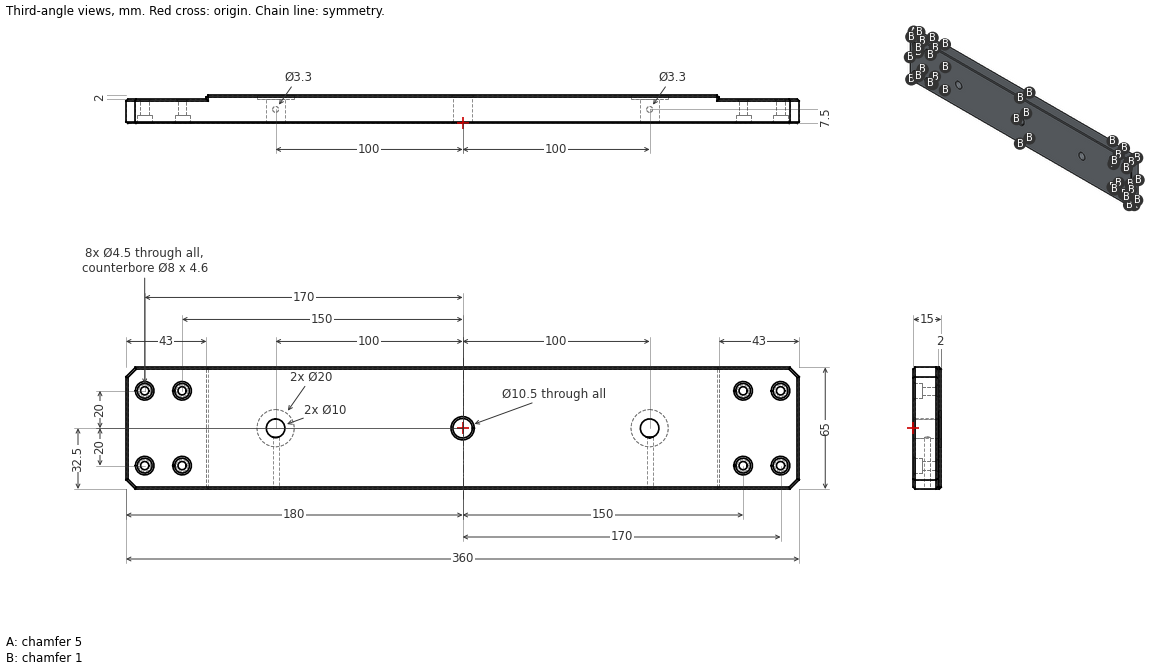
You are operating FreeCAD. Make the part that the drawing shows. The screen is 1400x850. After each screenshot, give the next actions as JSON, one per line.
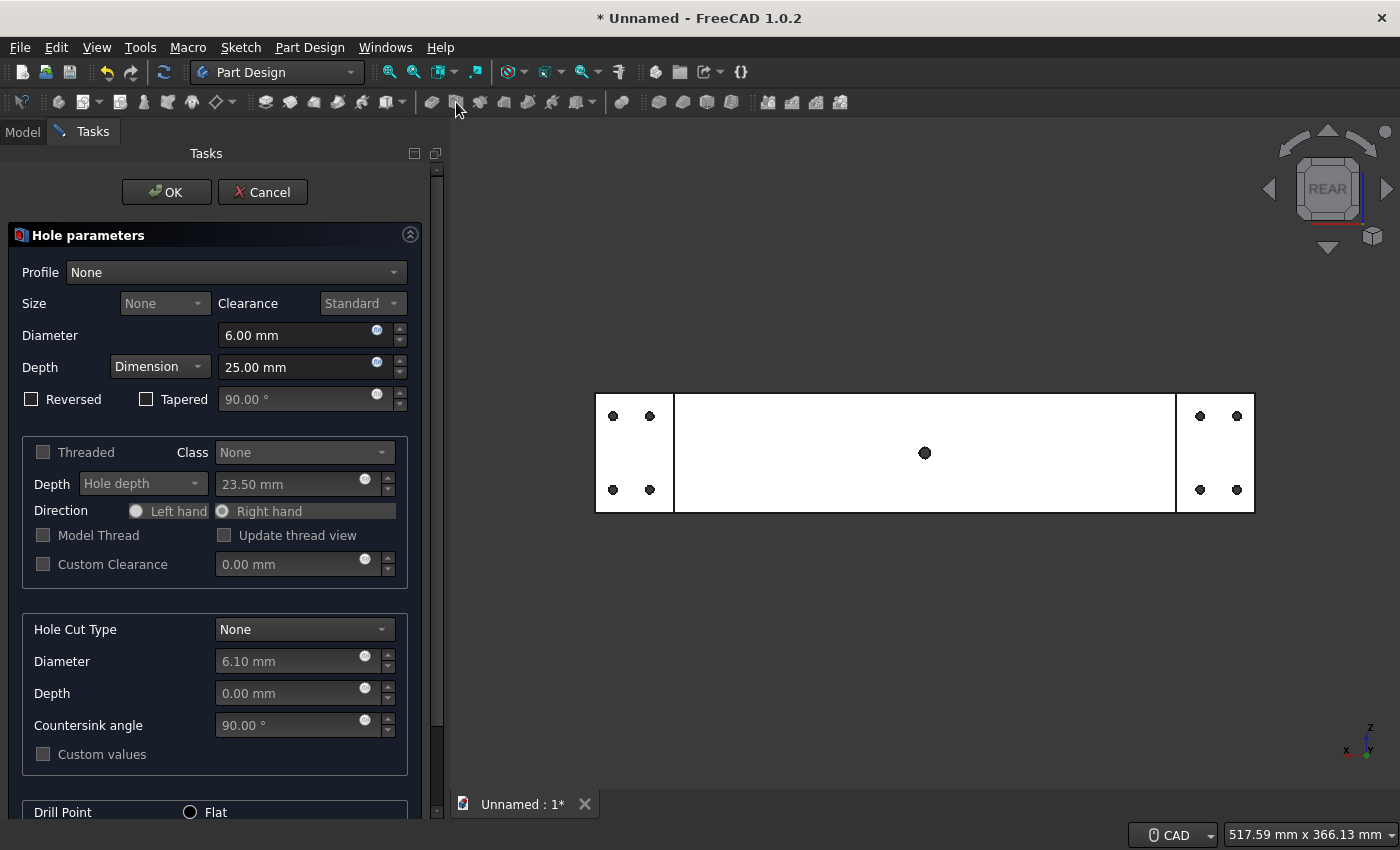
{"action": "triple_click", "coordinate": [305, 335]}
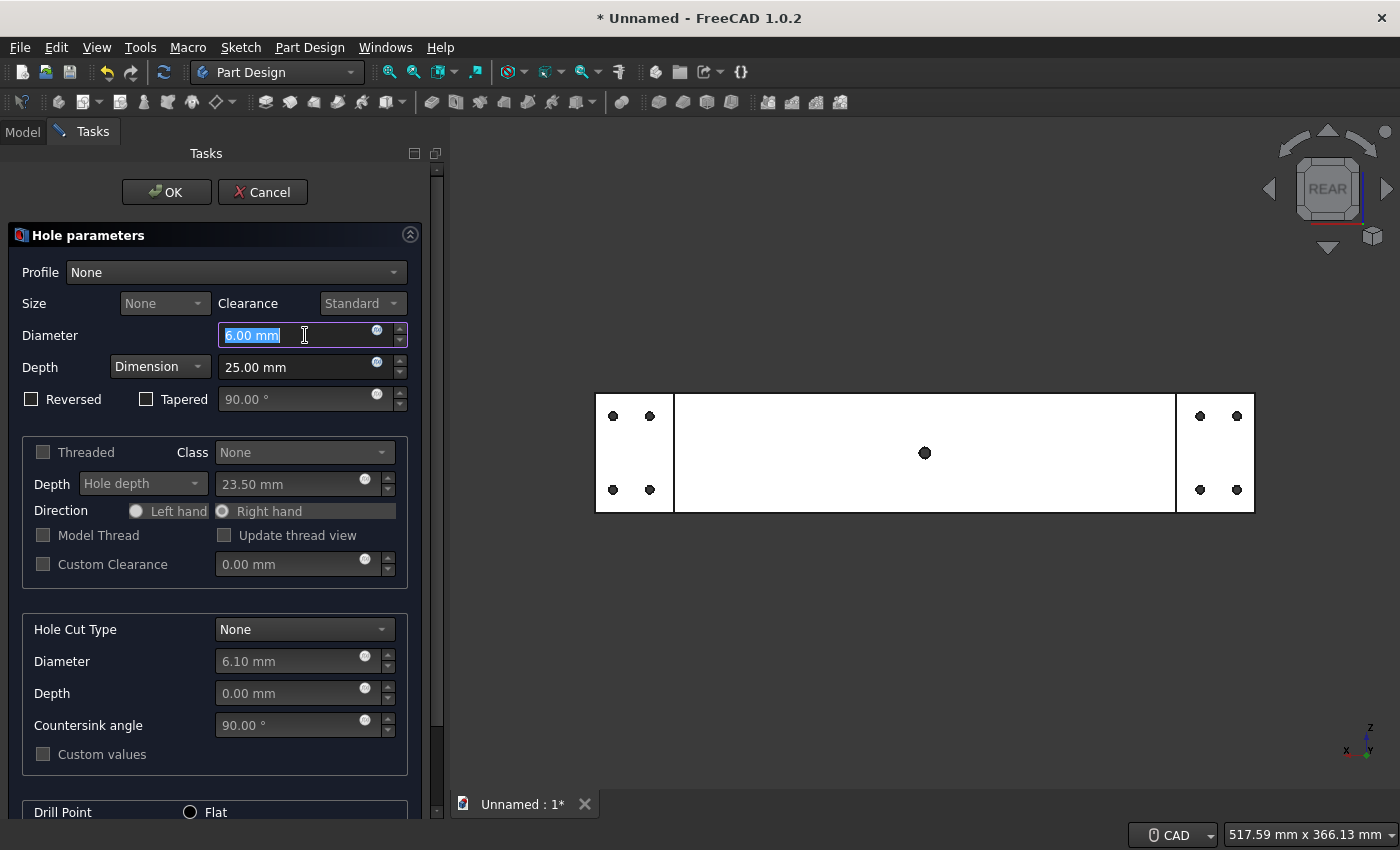
{"action": "type", "text": "10.5"}
{"action": "key", "text": "Tab"}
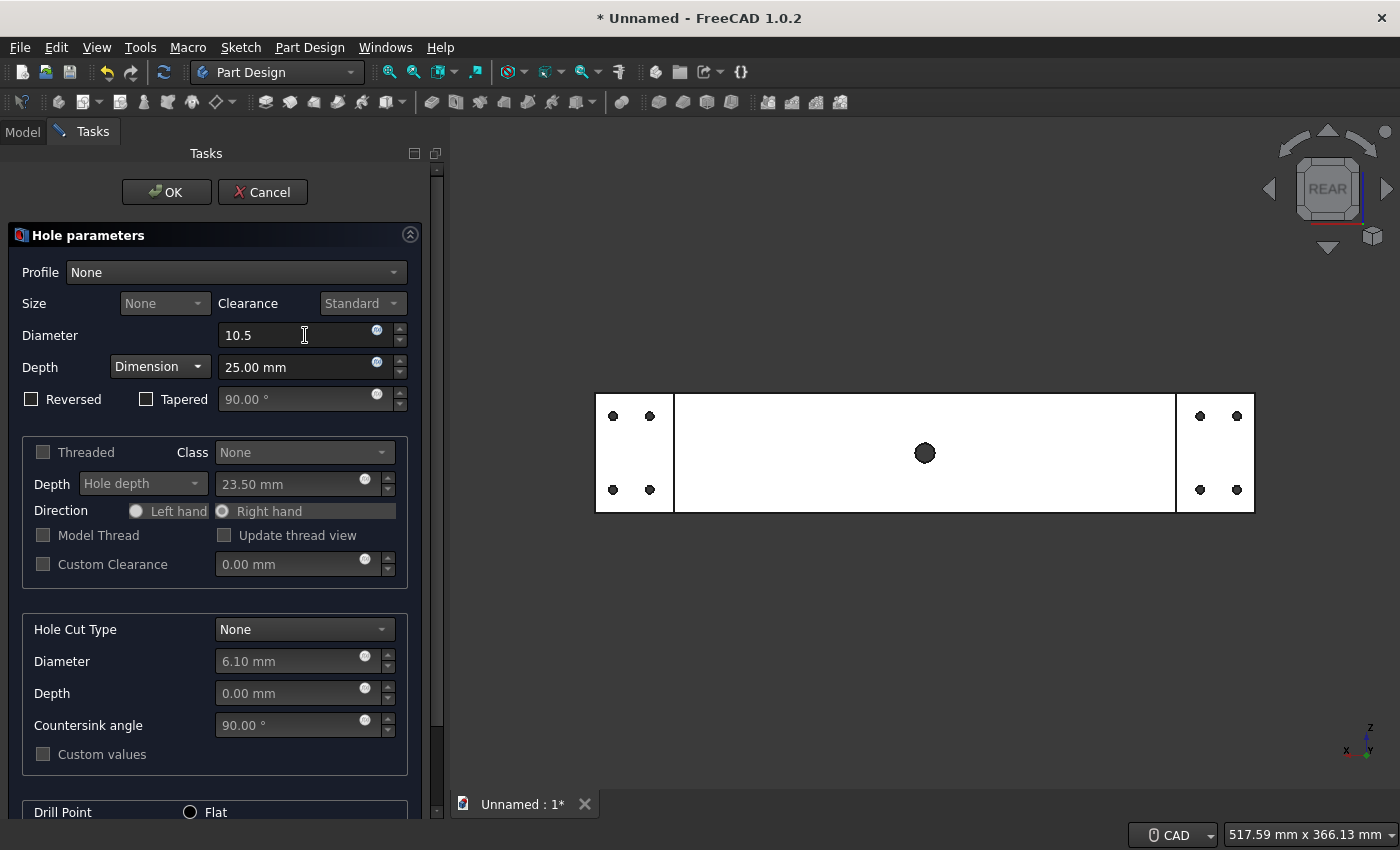
{"action": "left_click", "coordinate": [161, 366]}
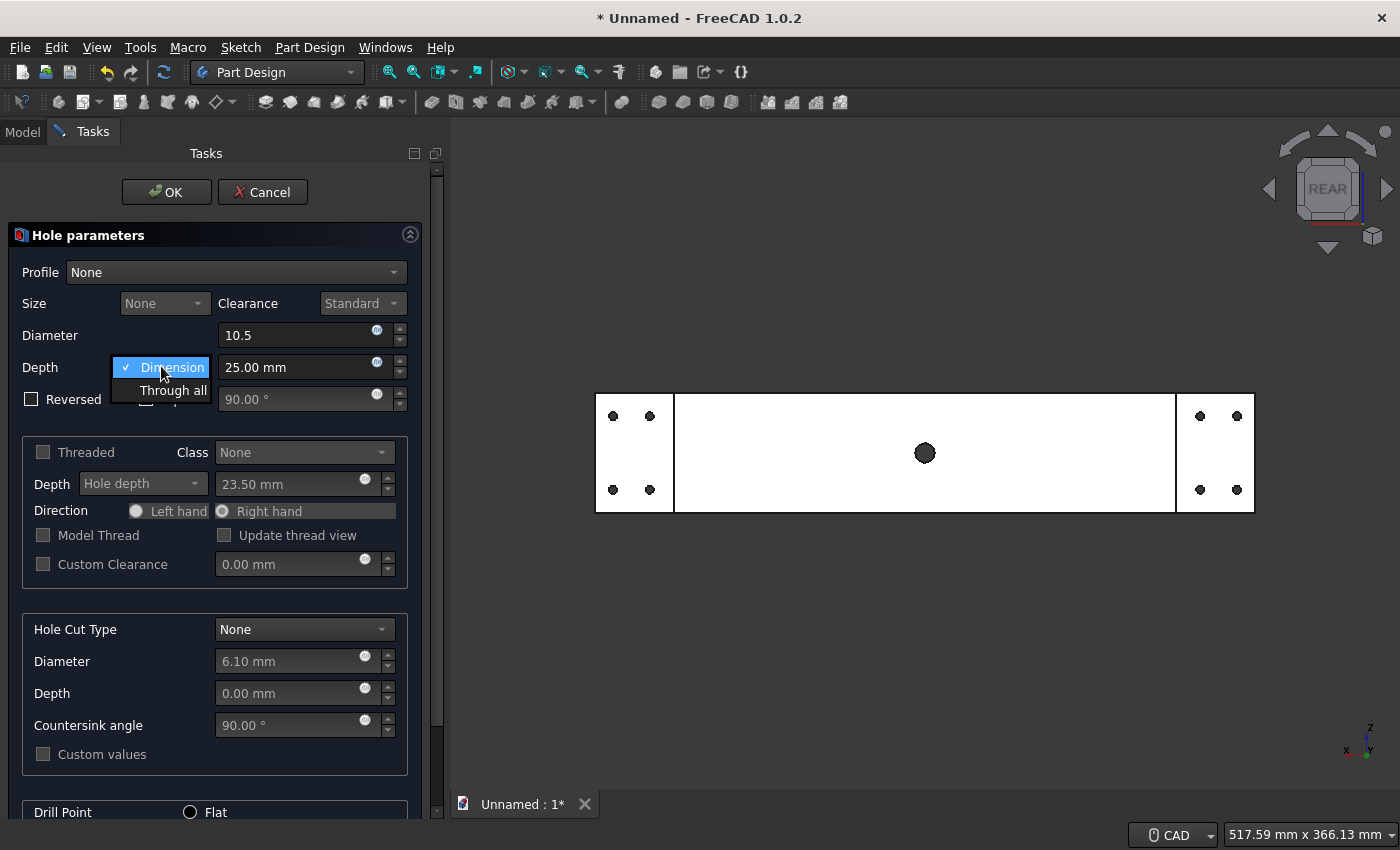
{"action": "left_click", "coordinate": [160, 390]}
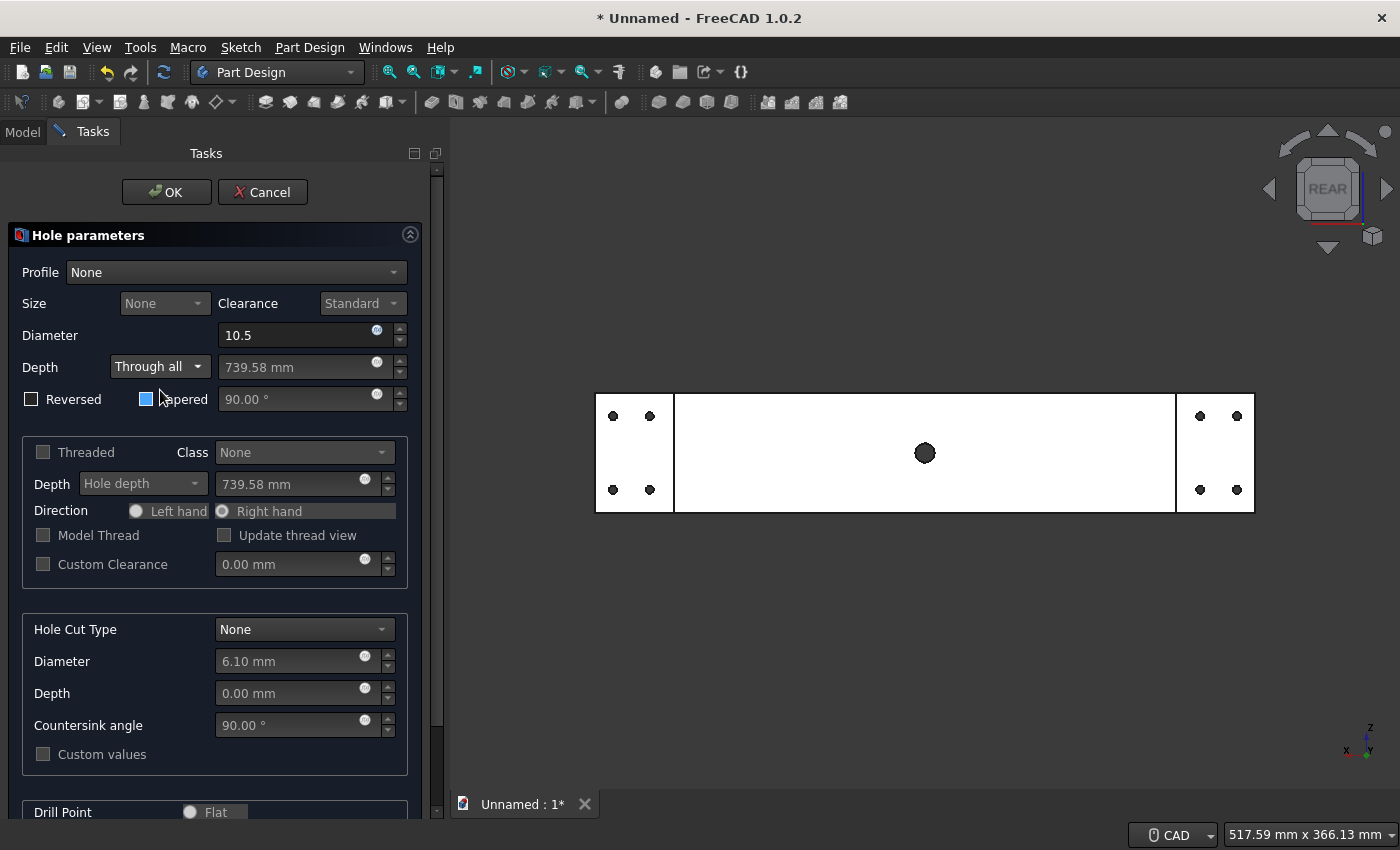
{"action": "left_click", "coordinate": [167, 192]}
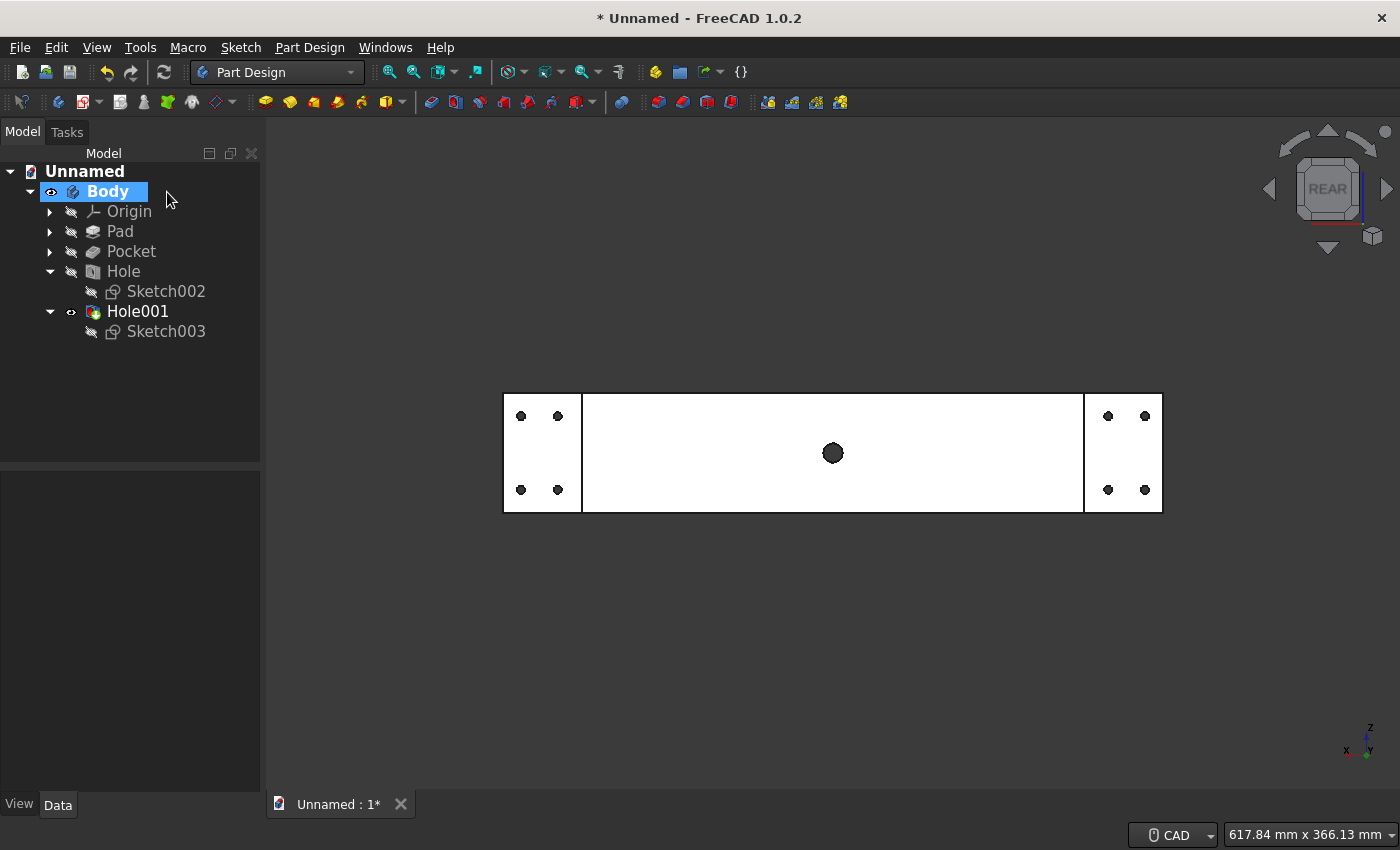
{"action": "key", "text": "0"}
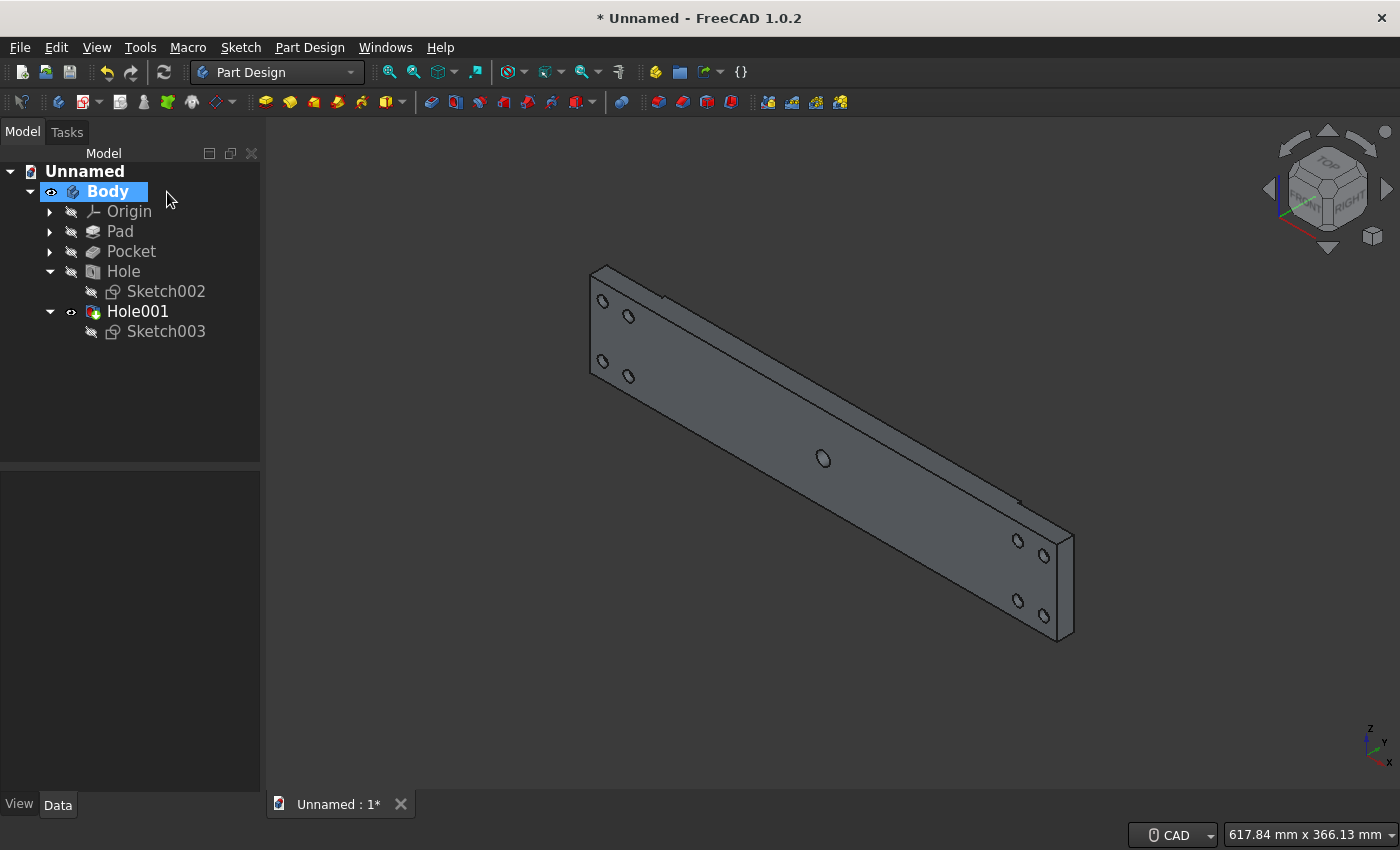
{"action": "left_click", "coordinate": [1065, 539]}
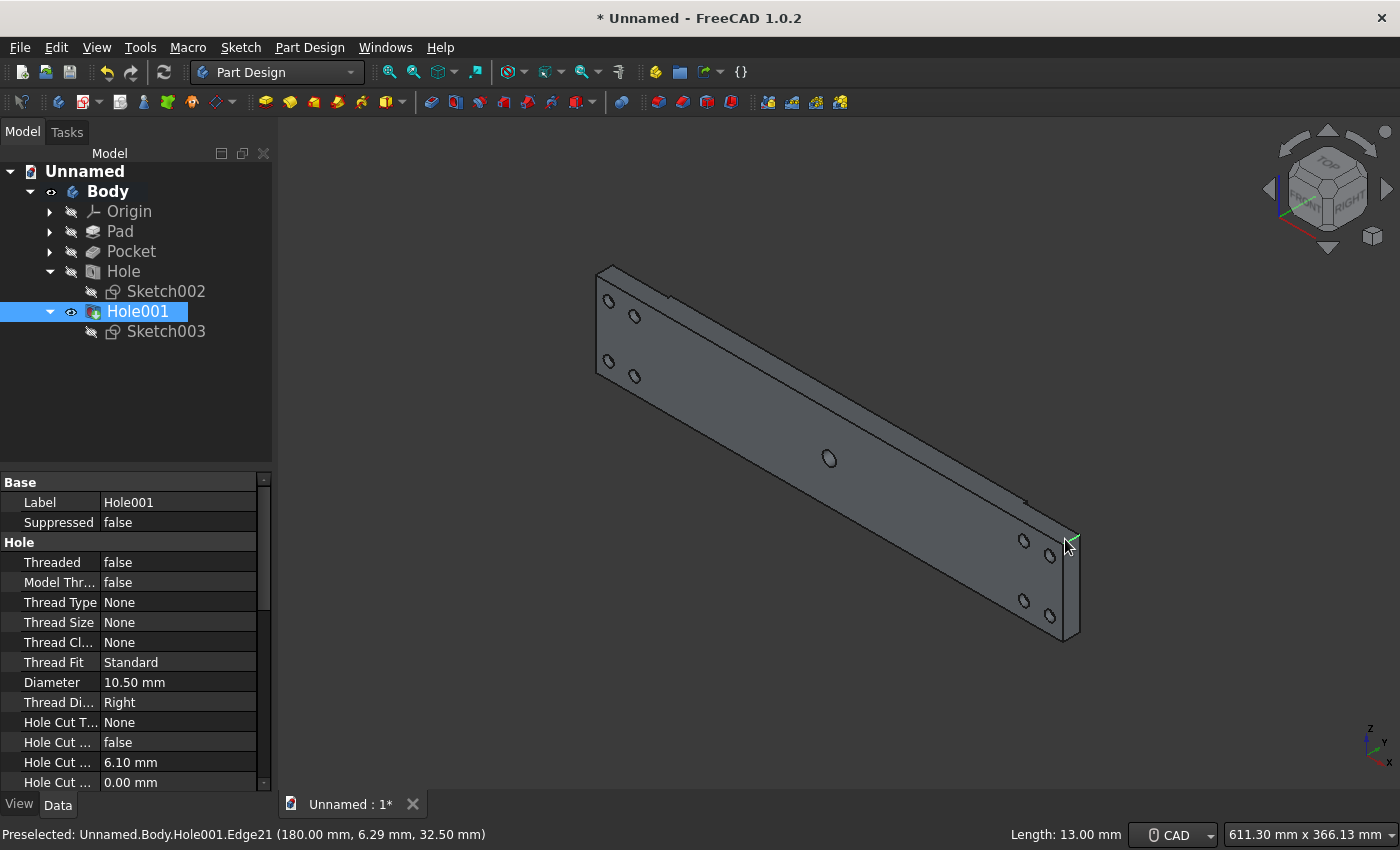
{"action": "key", "text": "2"}